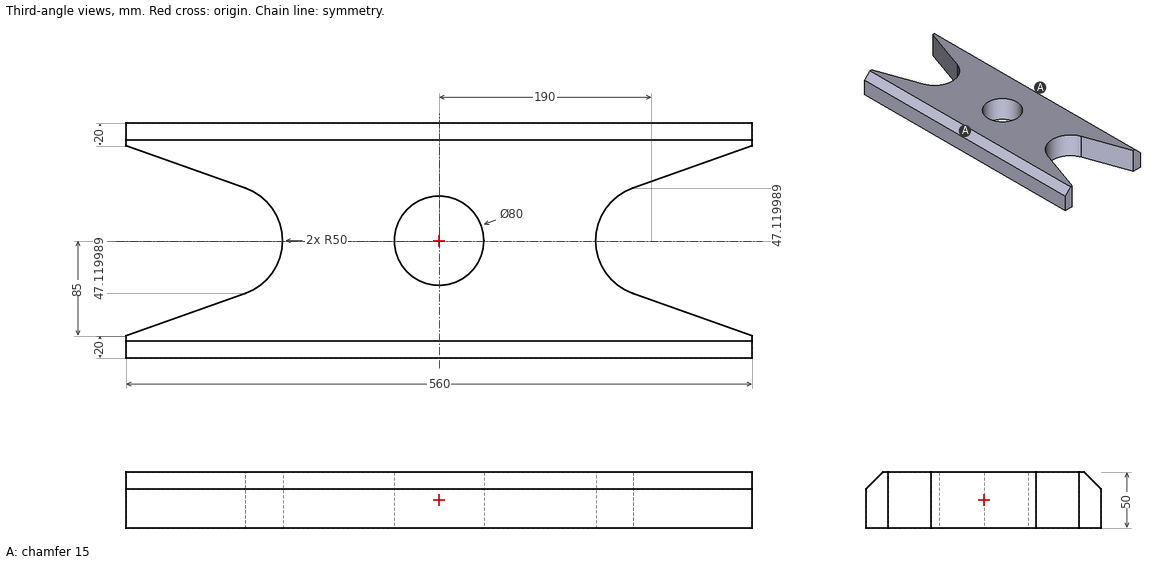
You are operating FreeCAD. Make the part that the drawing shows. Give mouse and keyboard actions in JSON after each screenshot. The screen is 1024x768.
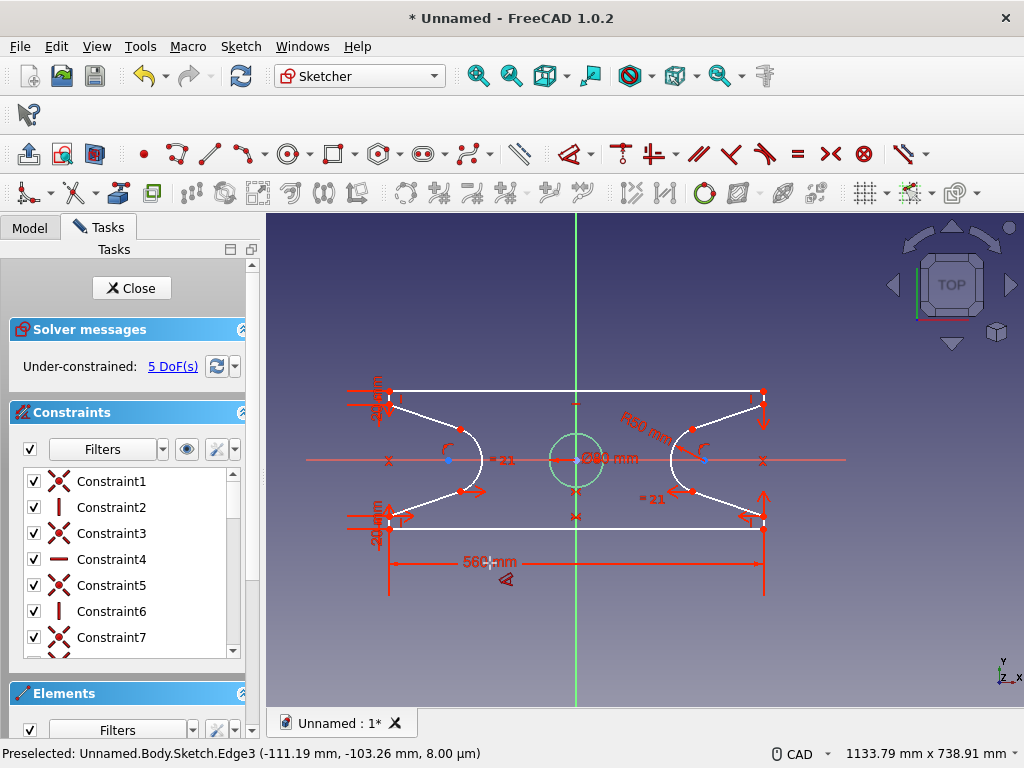
{"action": "left_click", "coordinate": [389, 516]}
{"action": "left_click", "coordinate": [355, 488]}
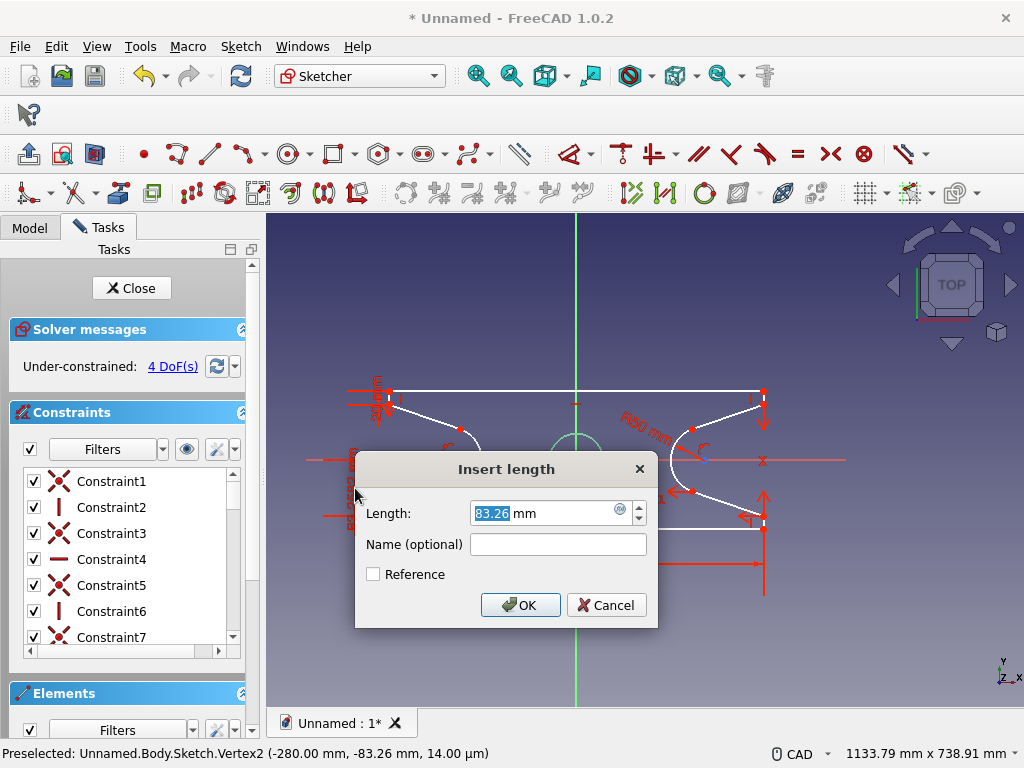
{"action": "type", "text": "85"}
{"action": "key", "text": "Return"}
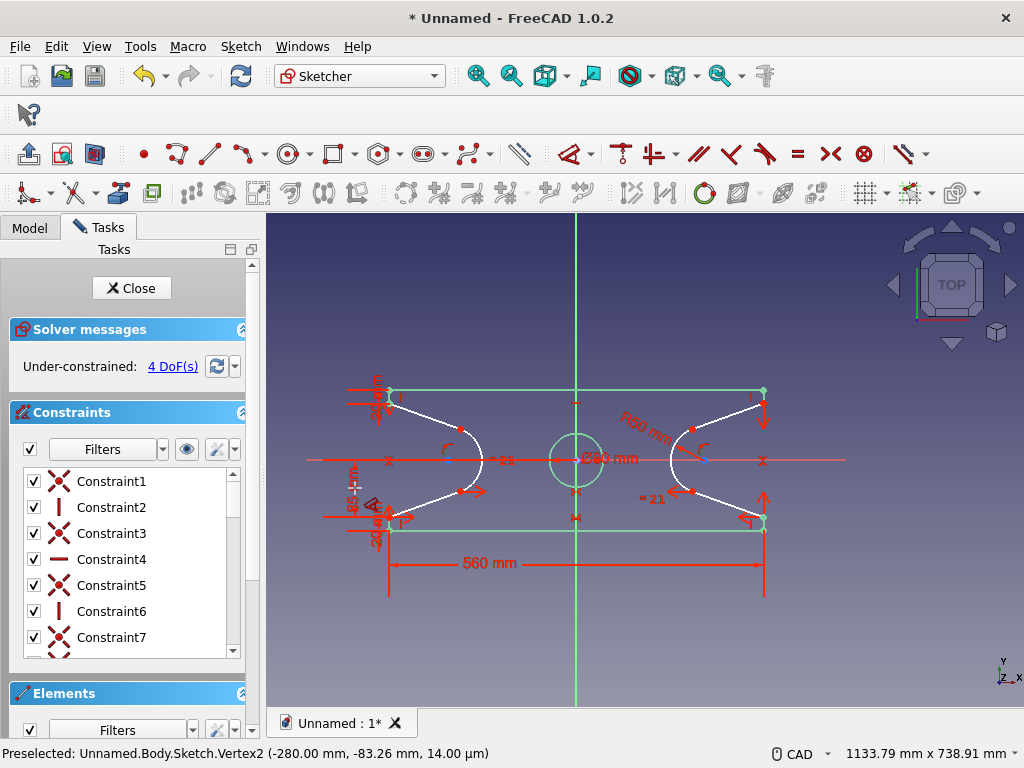
{"action": "left_click", "coordinate": [704, 460]}
{"action": "left_click", "coordinate": [640, 494]}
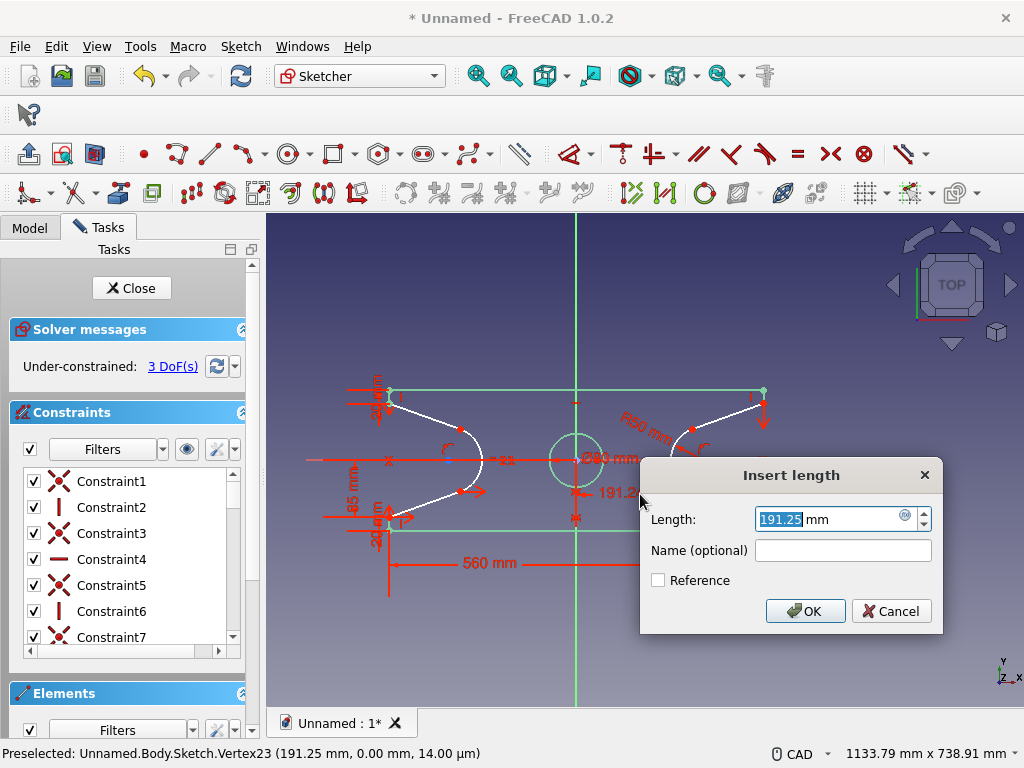
{"action": "type", "text": "190"}
{"action": "key", "text": "Return"}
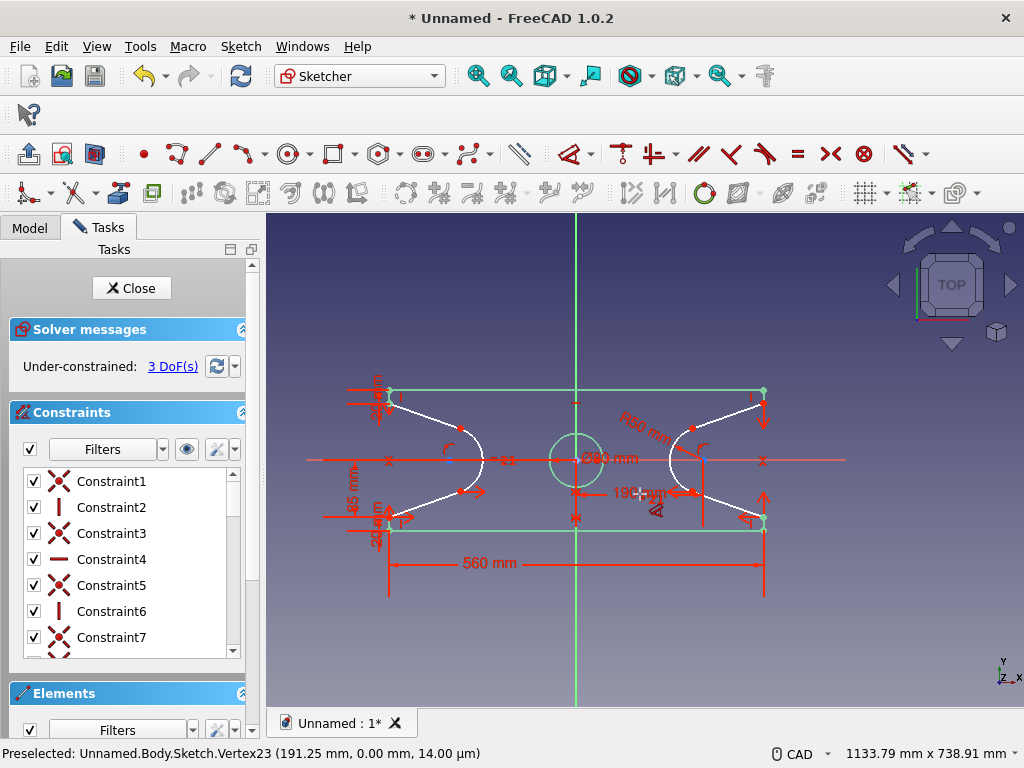
{"action": "scroll", "coordinate": [460, 492], "scroll_direction": "up", "scroll_amount": 2}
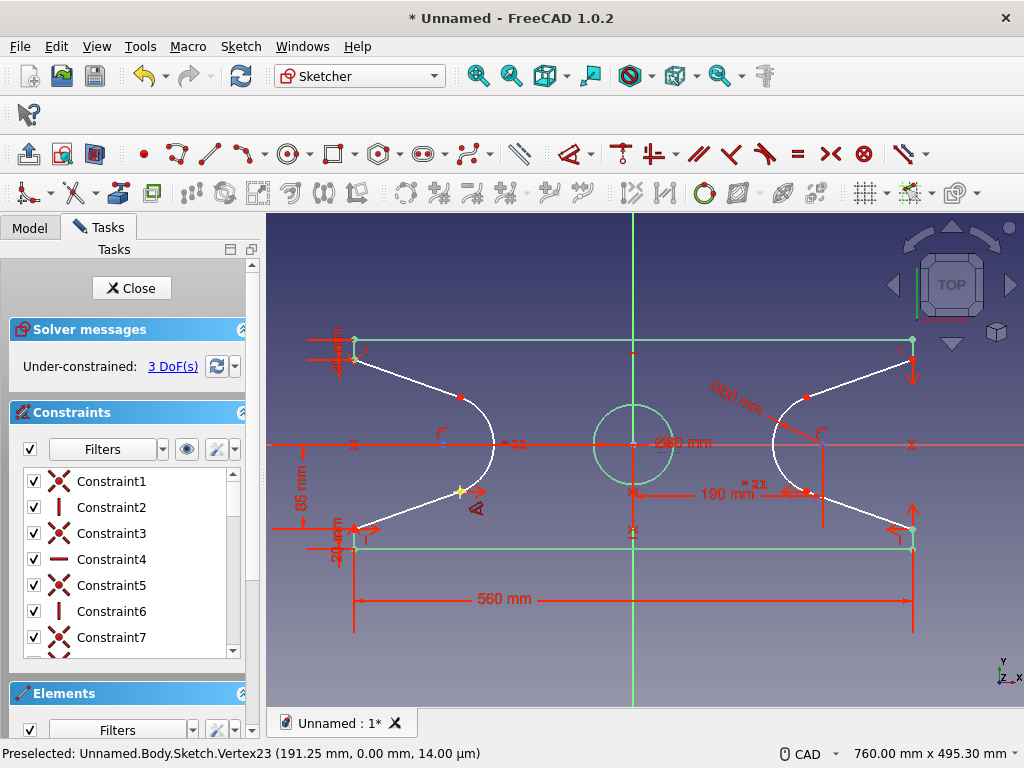
{"action": "left_click", "coordinate": [460, 492]}
{"action": "left_click", "coordinate": [426, 468]}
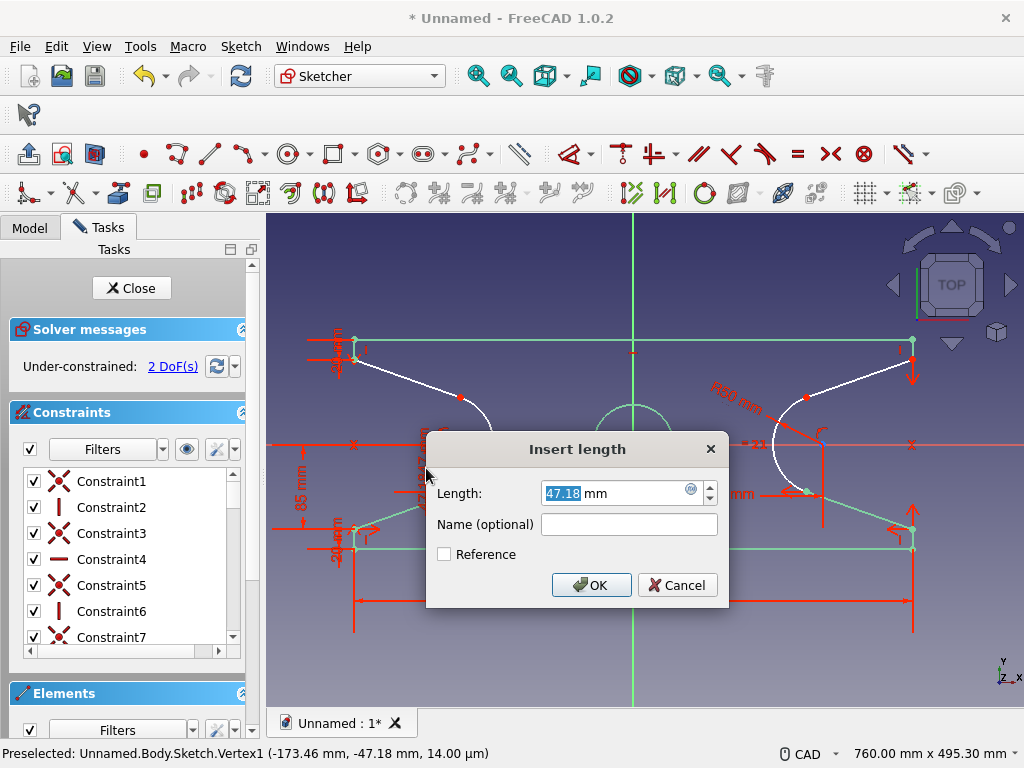
{"action": "type", "text": "47.119989"}
{"action": "key", "text": "Return"}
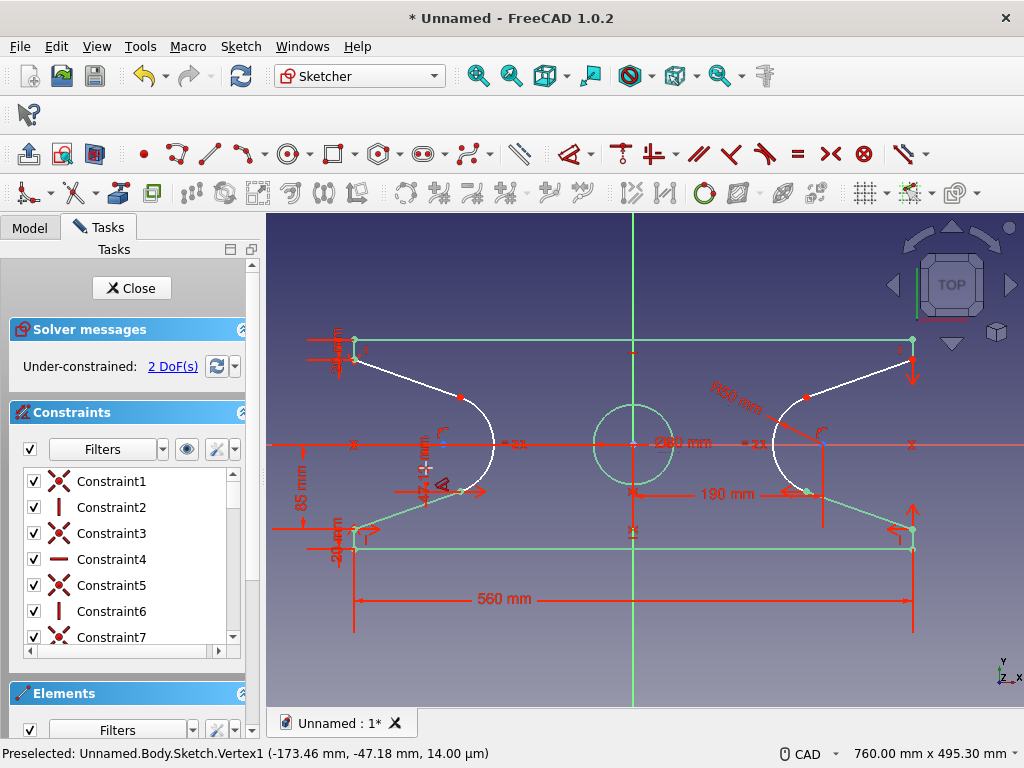
{"action": "left_click", "coordinate": [806, 398]}
{"action": "left_click", "coordinate": [840, 421]}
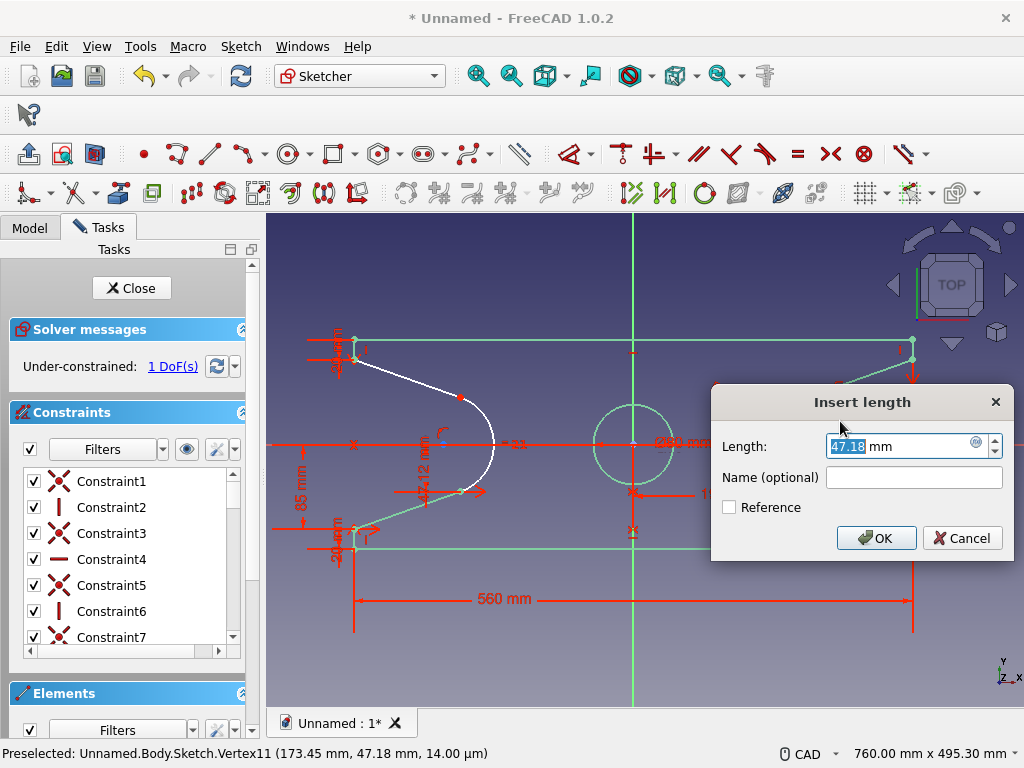
{"action": "type", "text": "47.119989"}
{"action": "key", "text": "Return"}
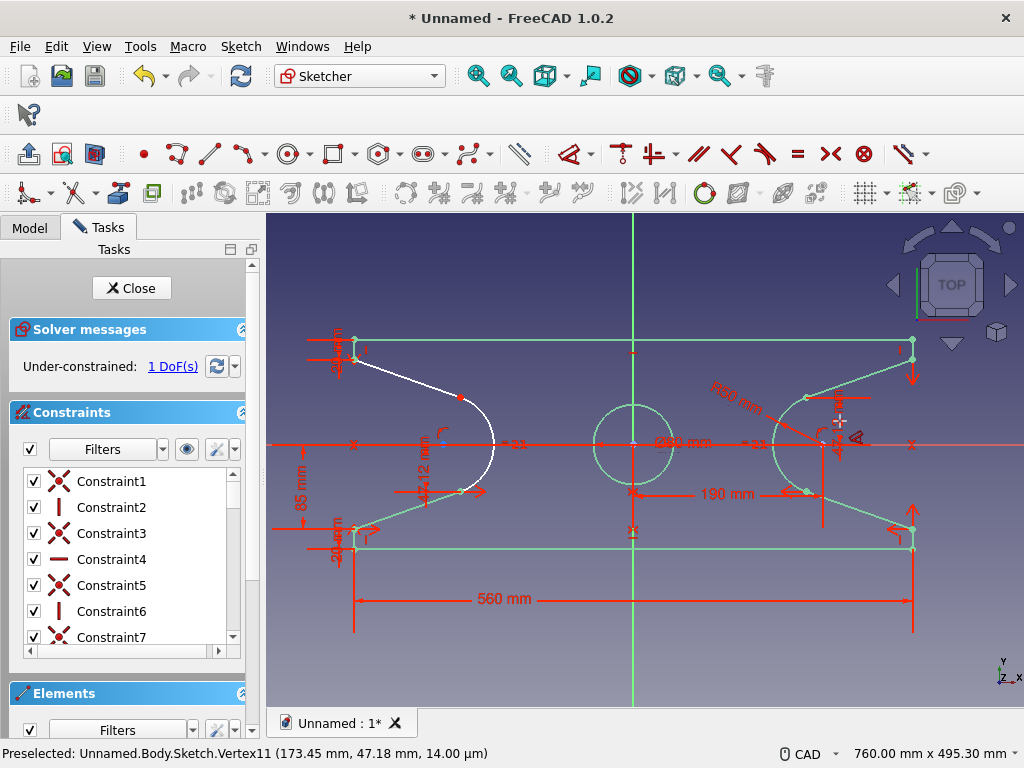
{"action": "left_click", "coordinate": [460, 398]}
{"action": "left_click", "coordinate": [426, 421]}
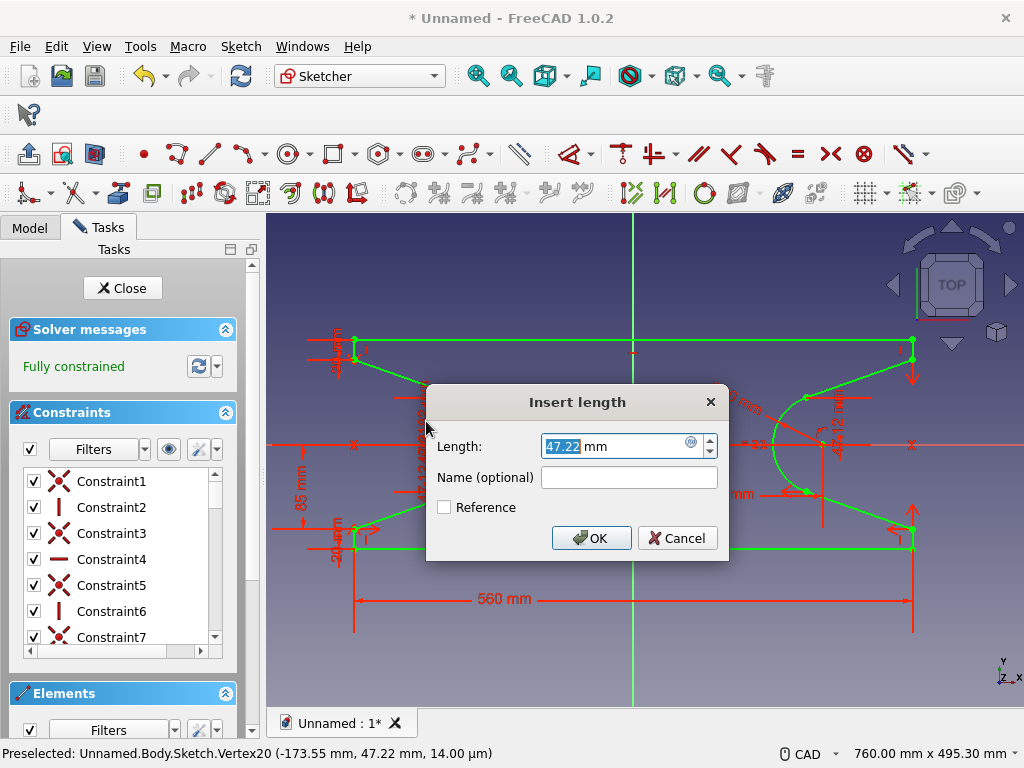
{"action": "type", "text": "47.119989"}
{"action": "key", "text": "Return"}
{"action": "key", "text": "Escape"}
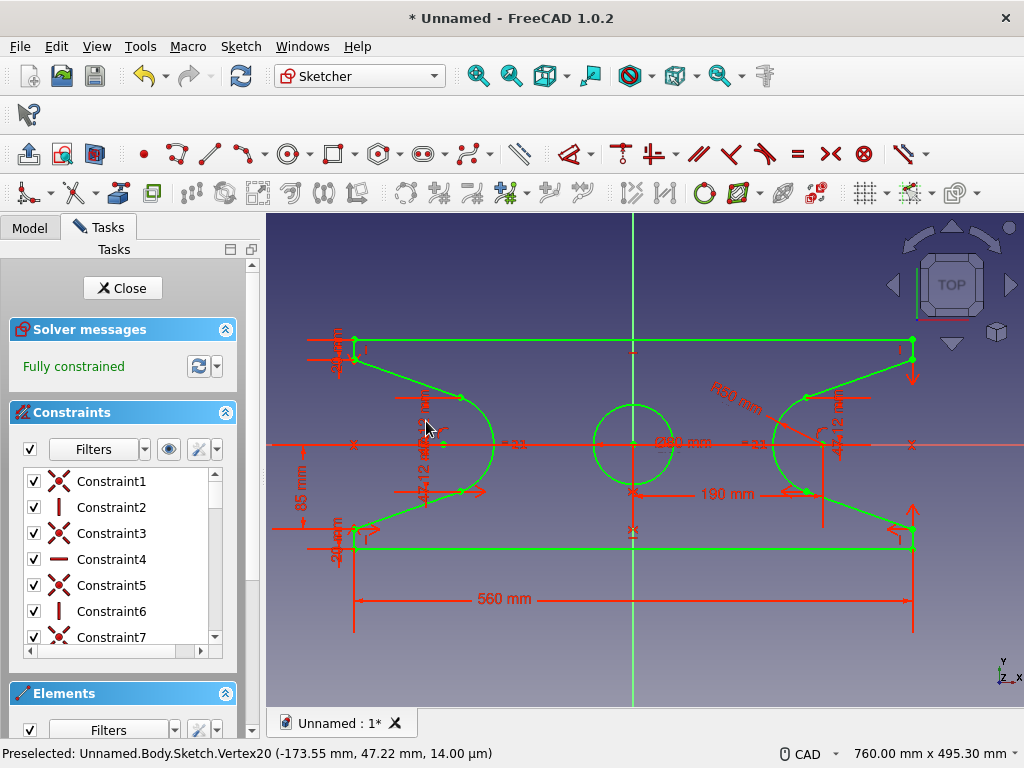
{"action": "left_click", "coordinate": [123, 288]}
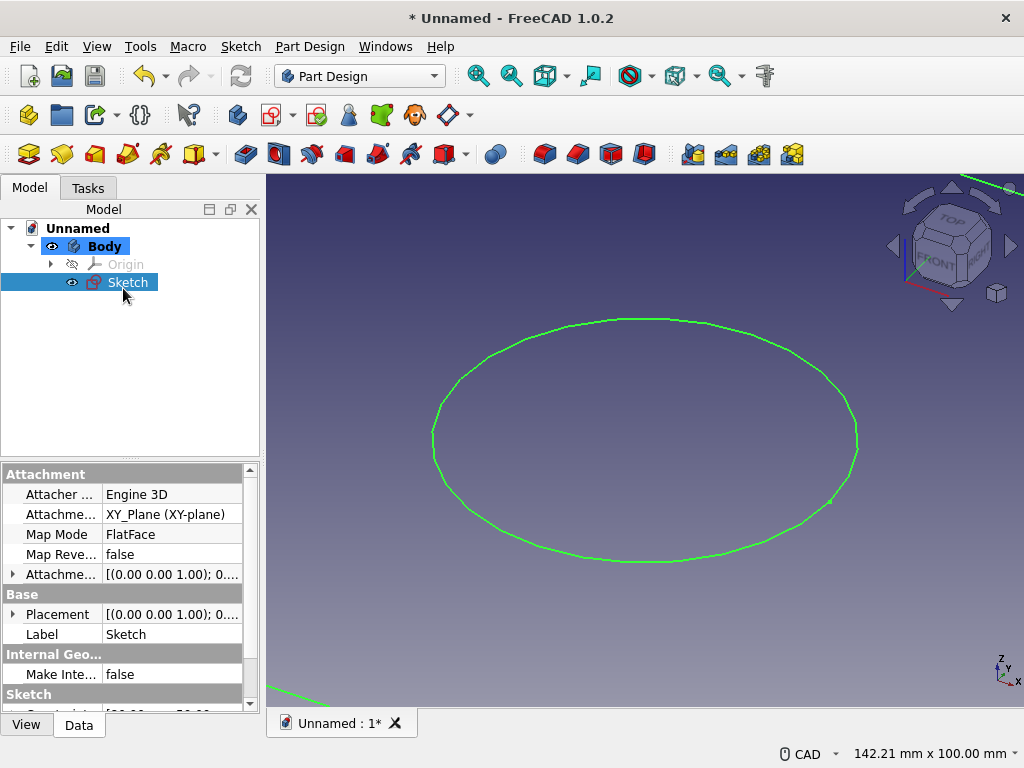
{"action": "left_click", "coordinate": [29, 154]}